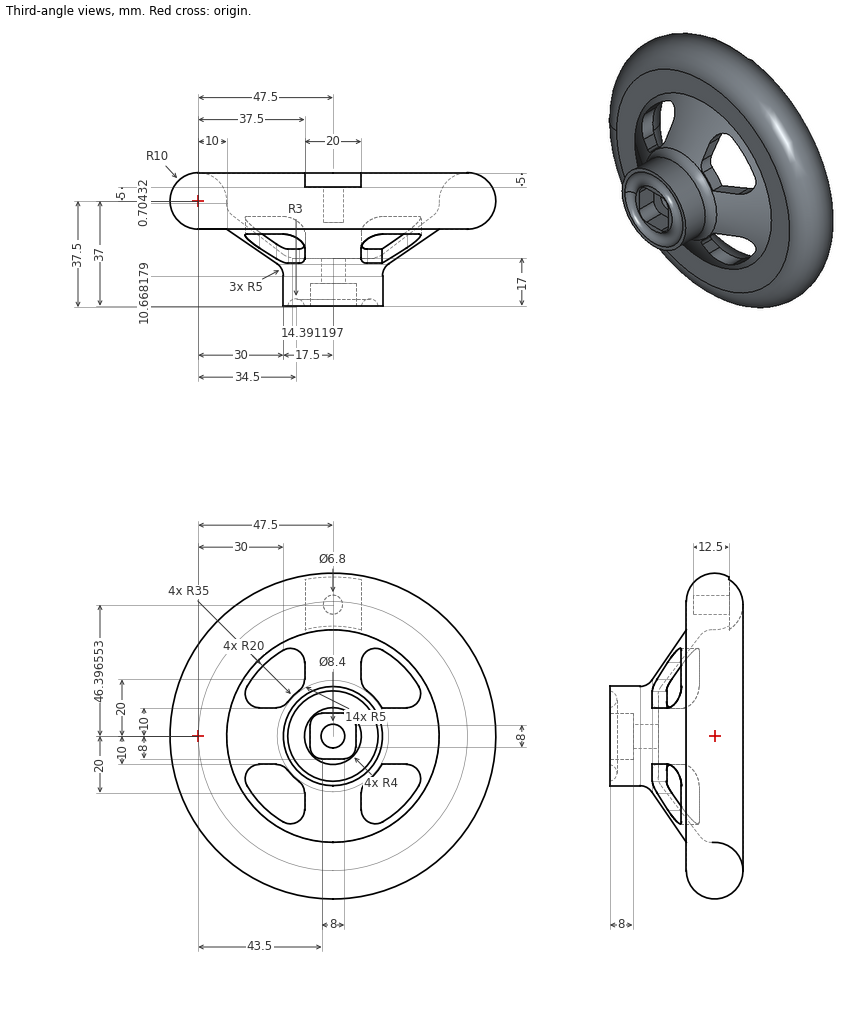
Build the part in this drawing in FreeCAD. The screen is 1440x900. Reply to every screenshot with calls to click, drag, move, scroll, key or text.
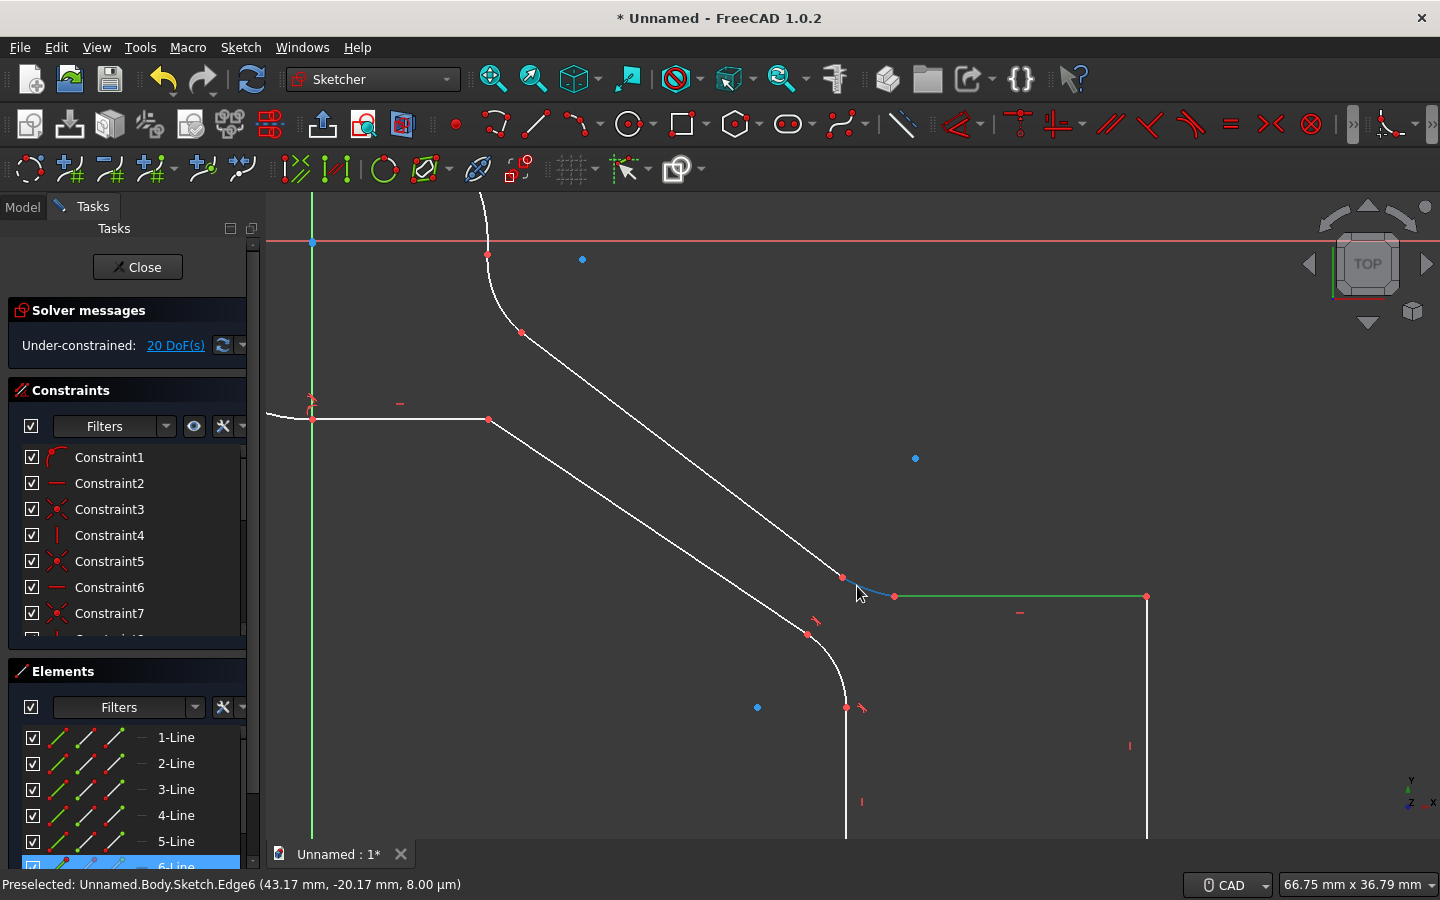
click(857, 585)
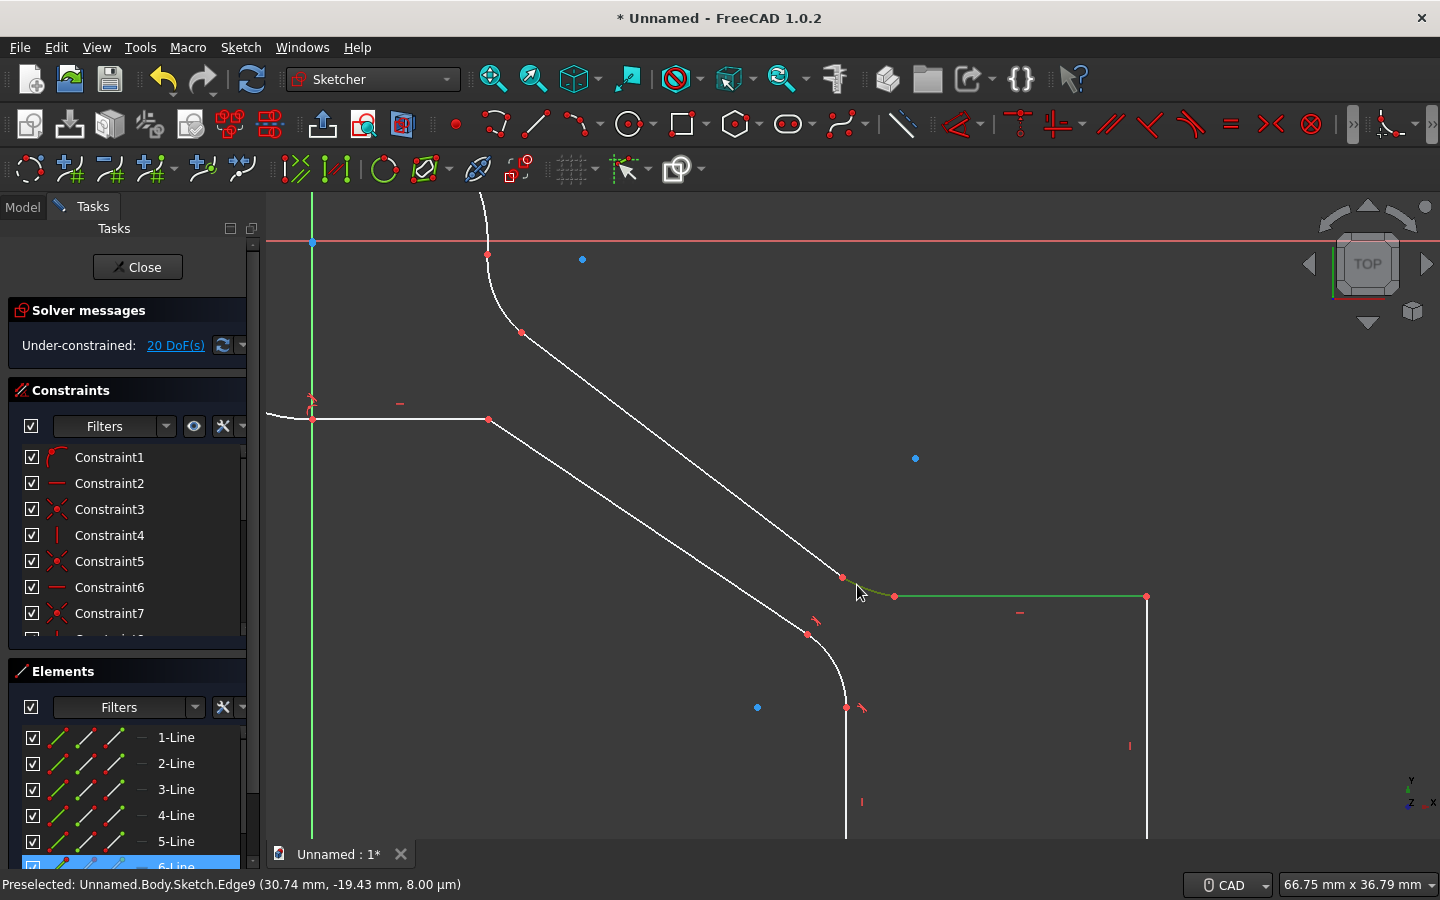
click(1192, 124)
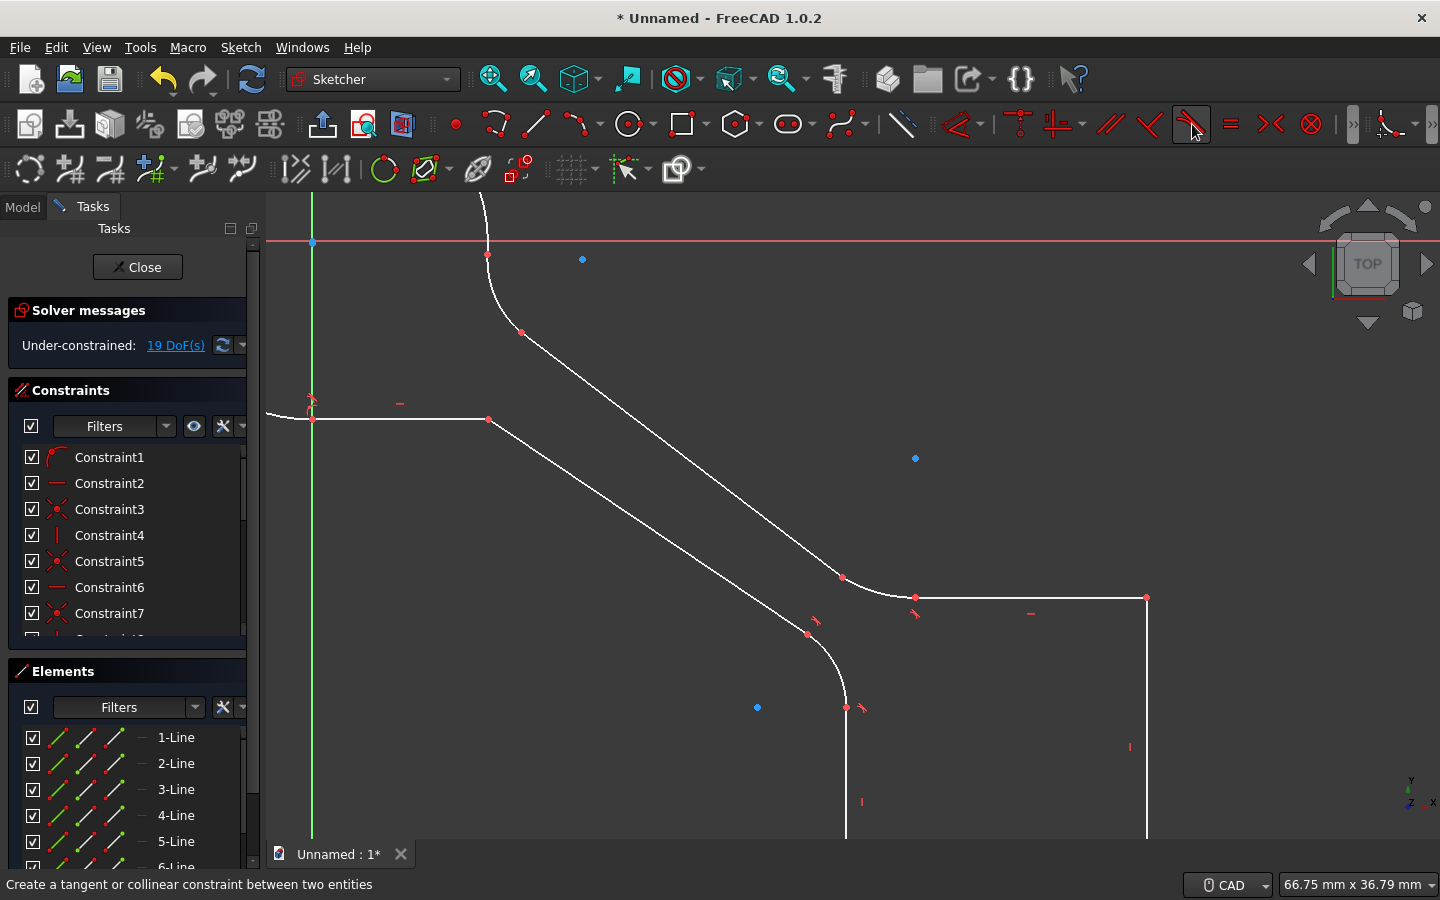
click(746, 504)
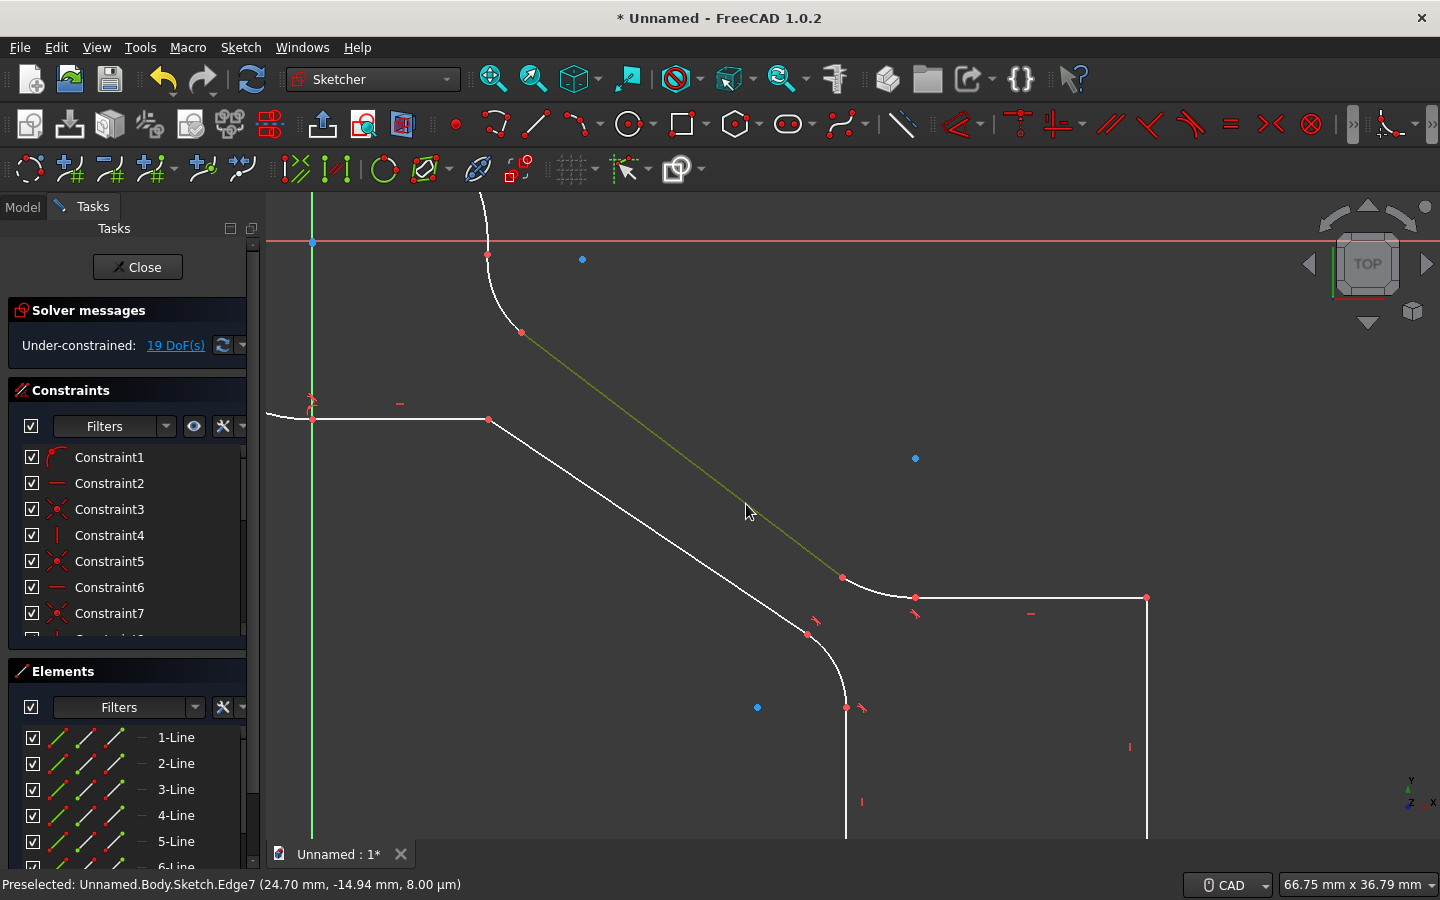
click(863, 588)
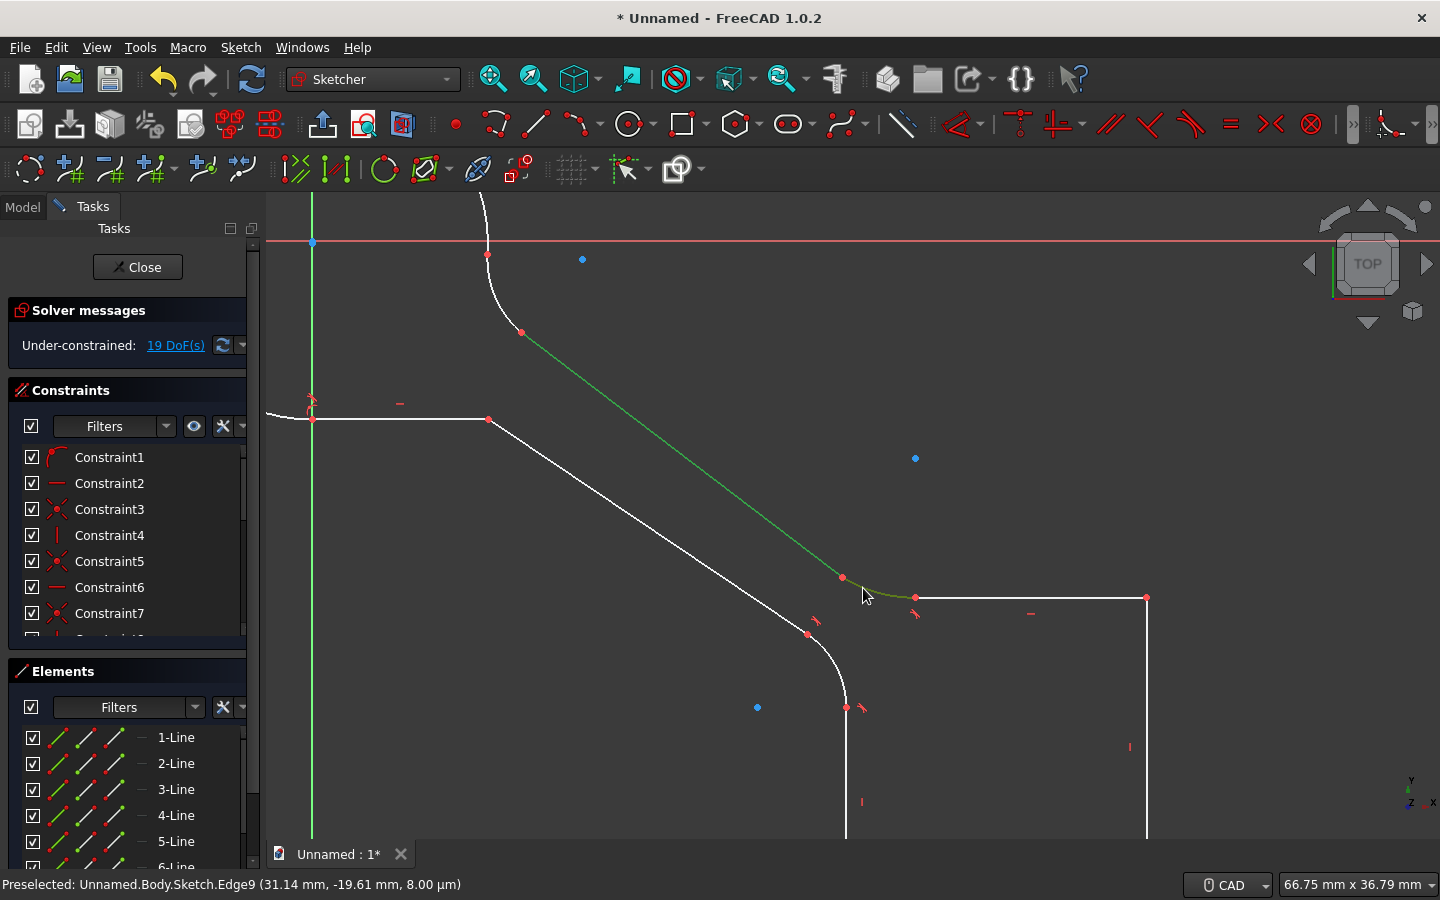
click(1192, 124)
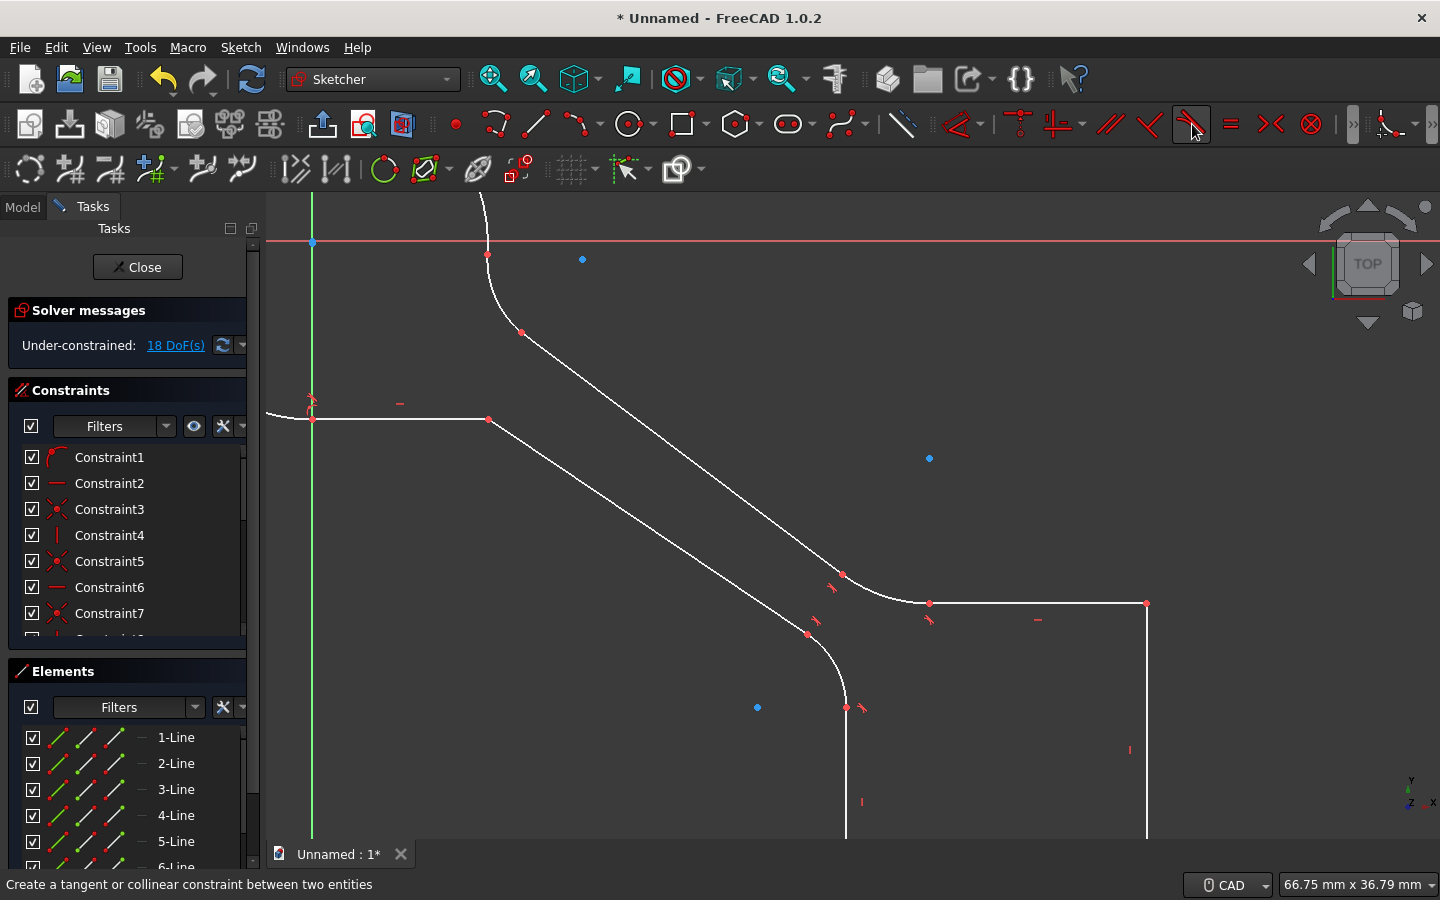
click(746, 502)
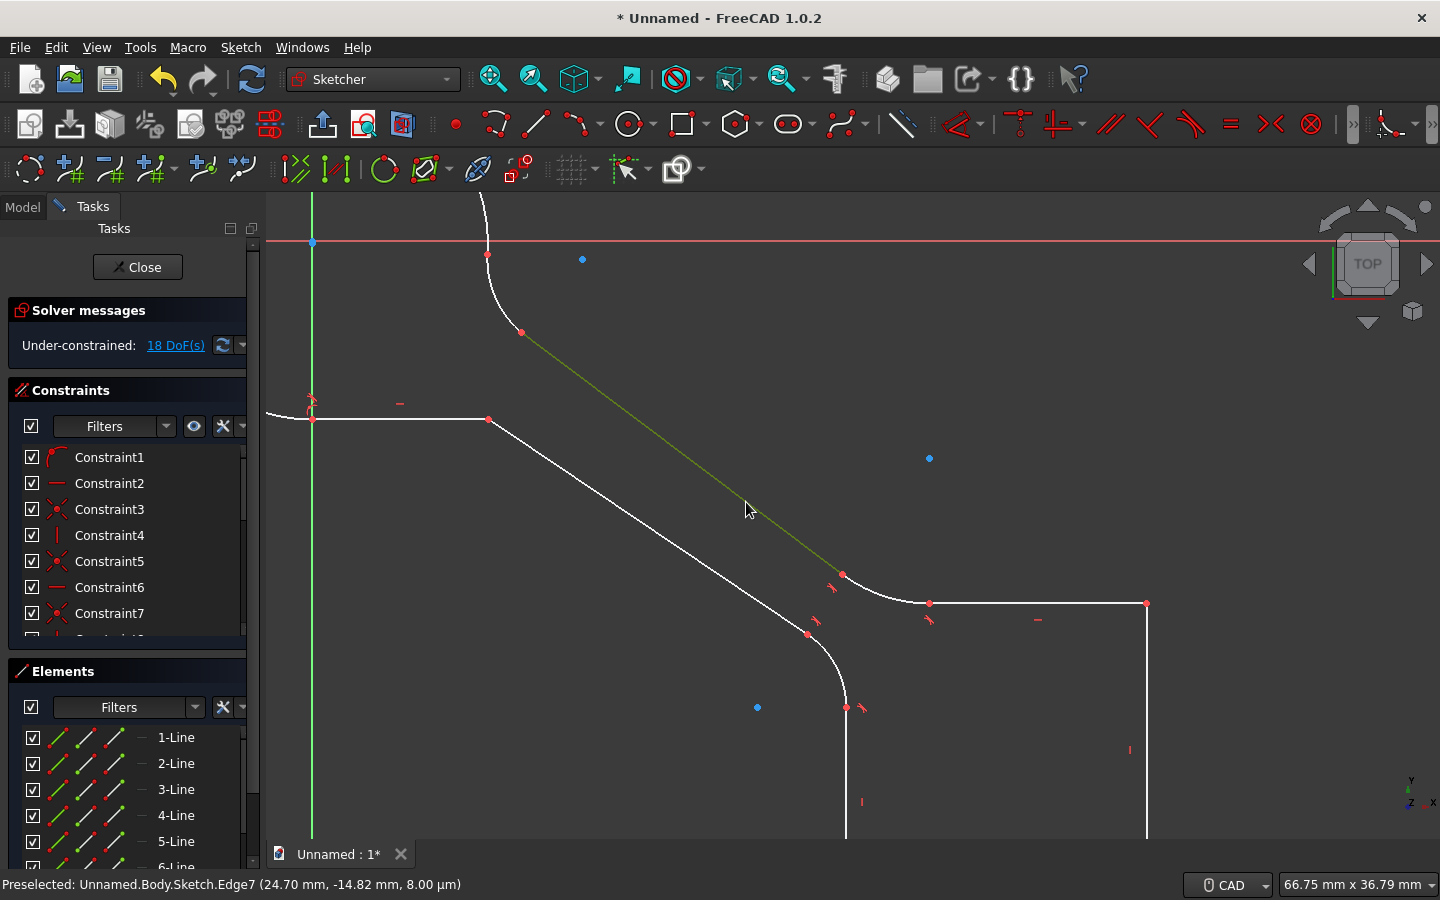
click(490, 281)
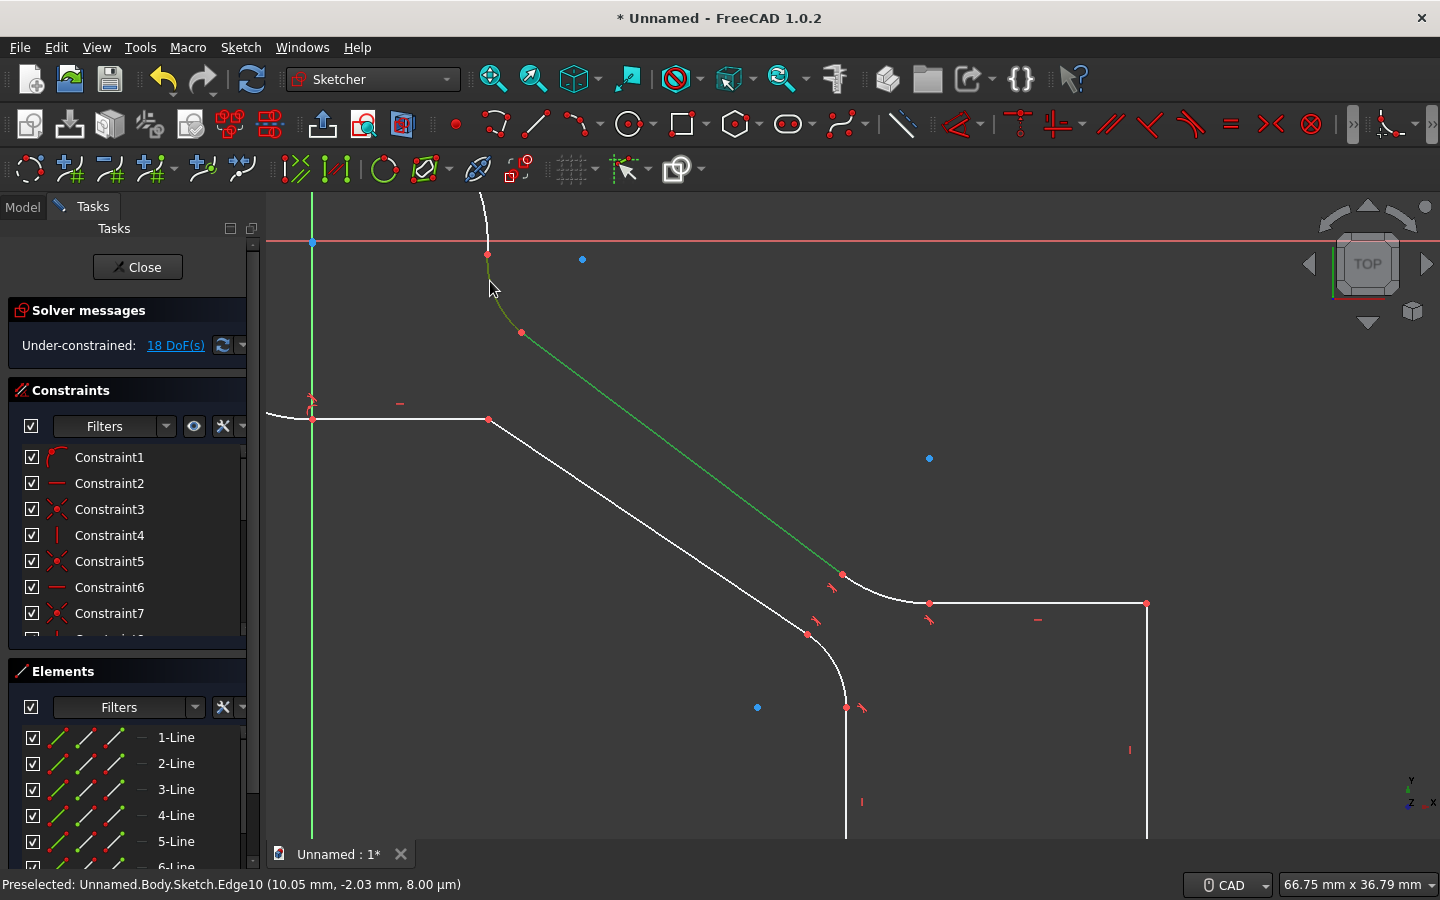
click(1192, 124)